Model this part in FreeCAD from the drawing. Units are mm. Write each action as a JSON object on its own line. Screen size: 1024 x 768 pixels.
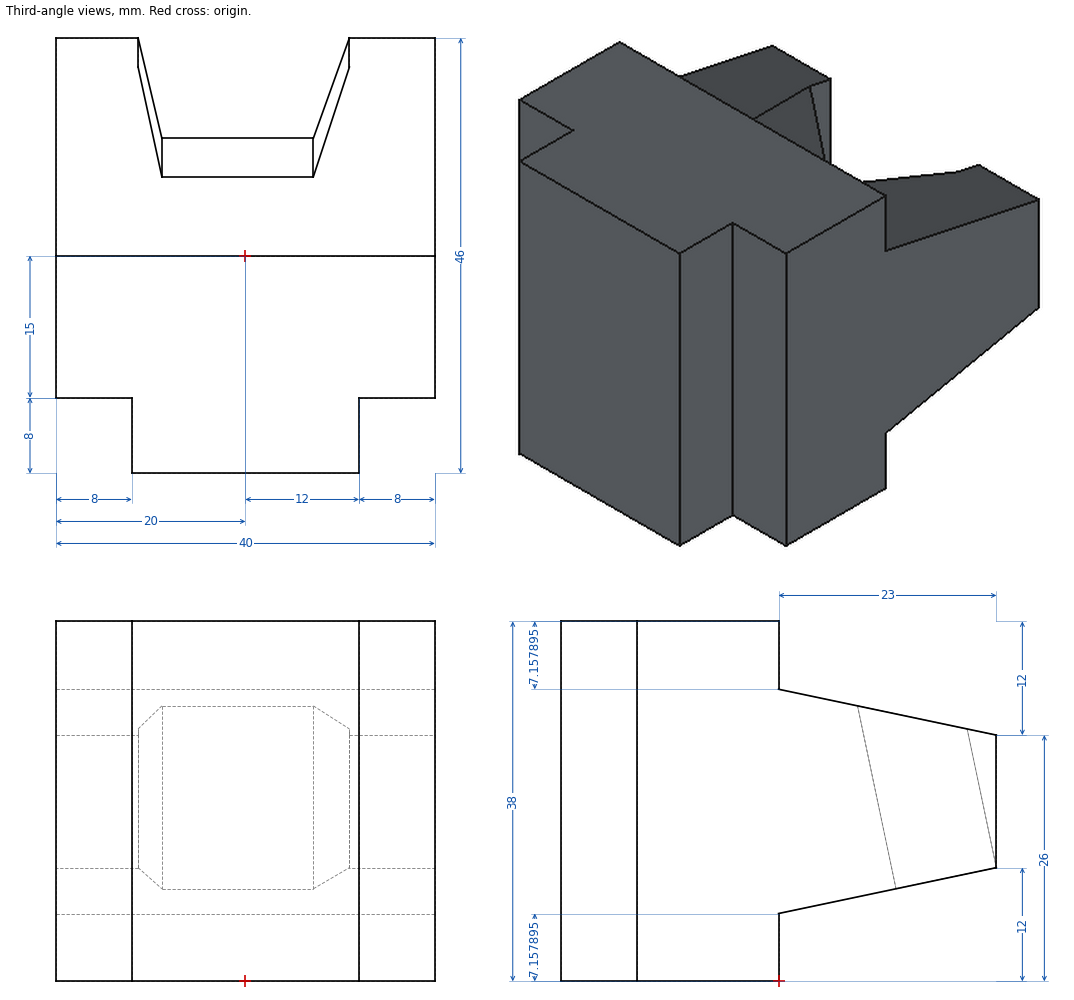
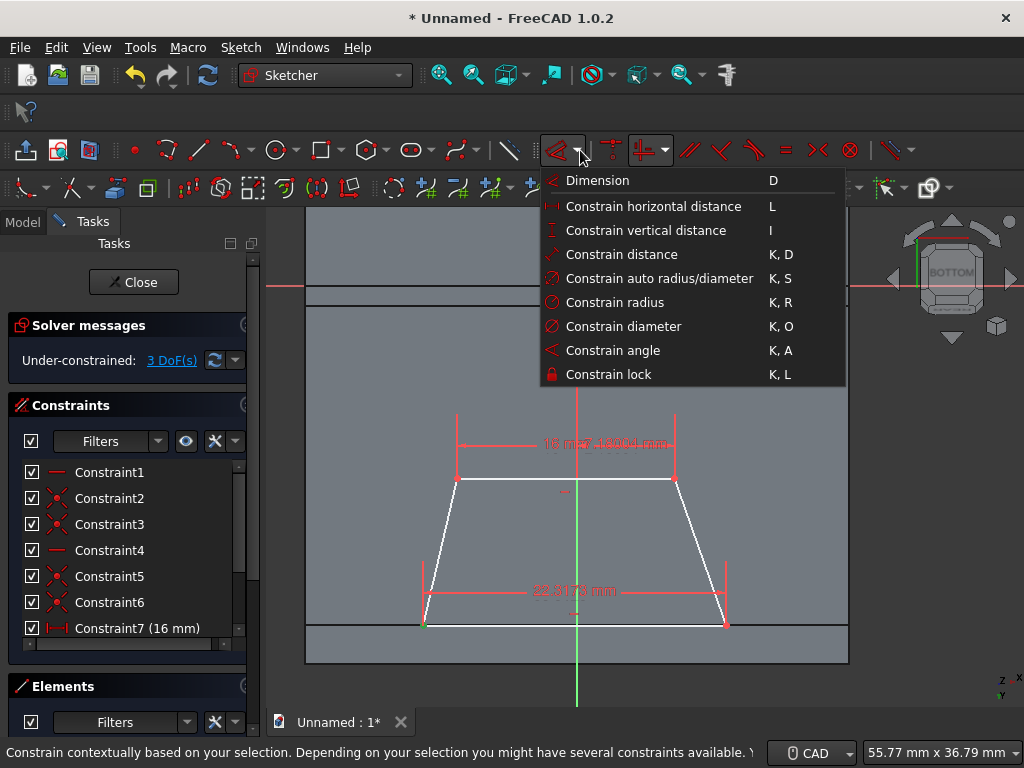
{"action": "left_click", "coordinate": [693, 206]}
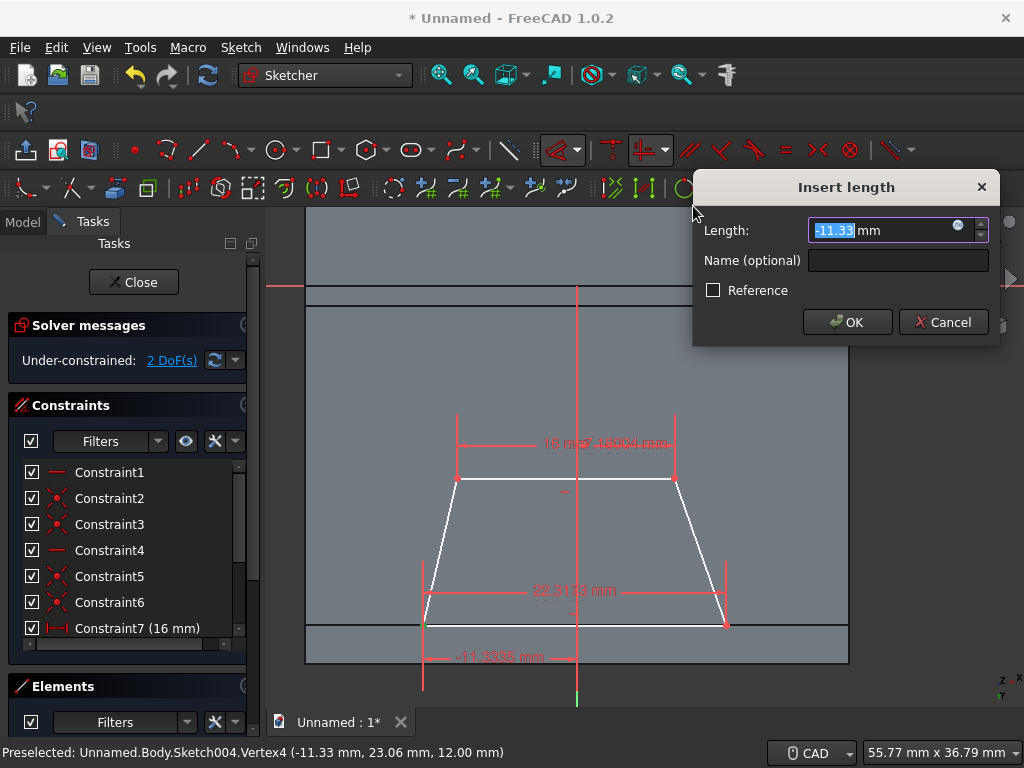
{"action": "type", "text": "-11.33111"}
{"action": "key", "text": "Return"}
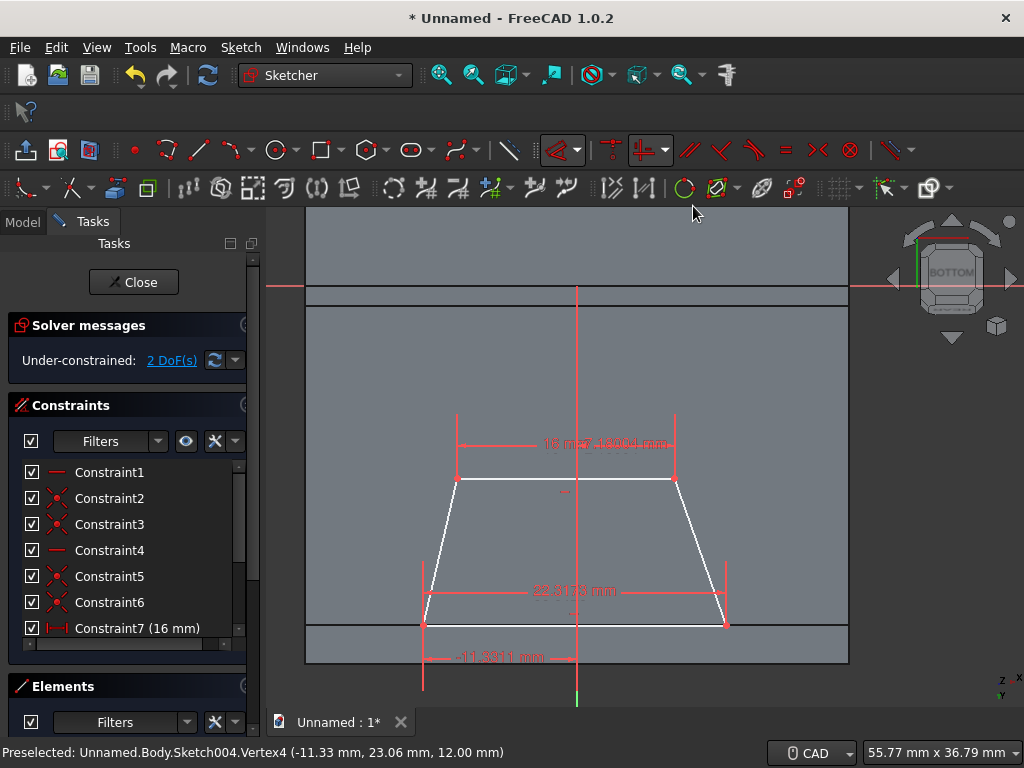
{"action": "left_click", "coordinate": [675, 479]}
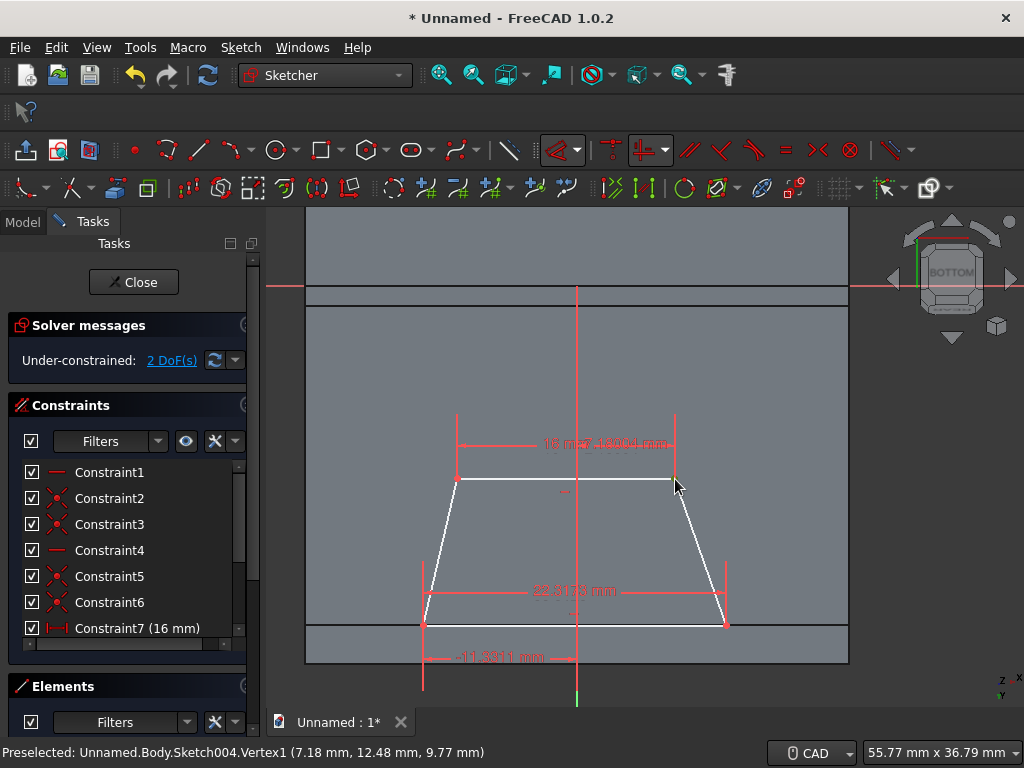
{"action": "key", "text": "i"}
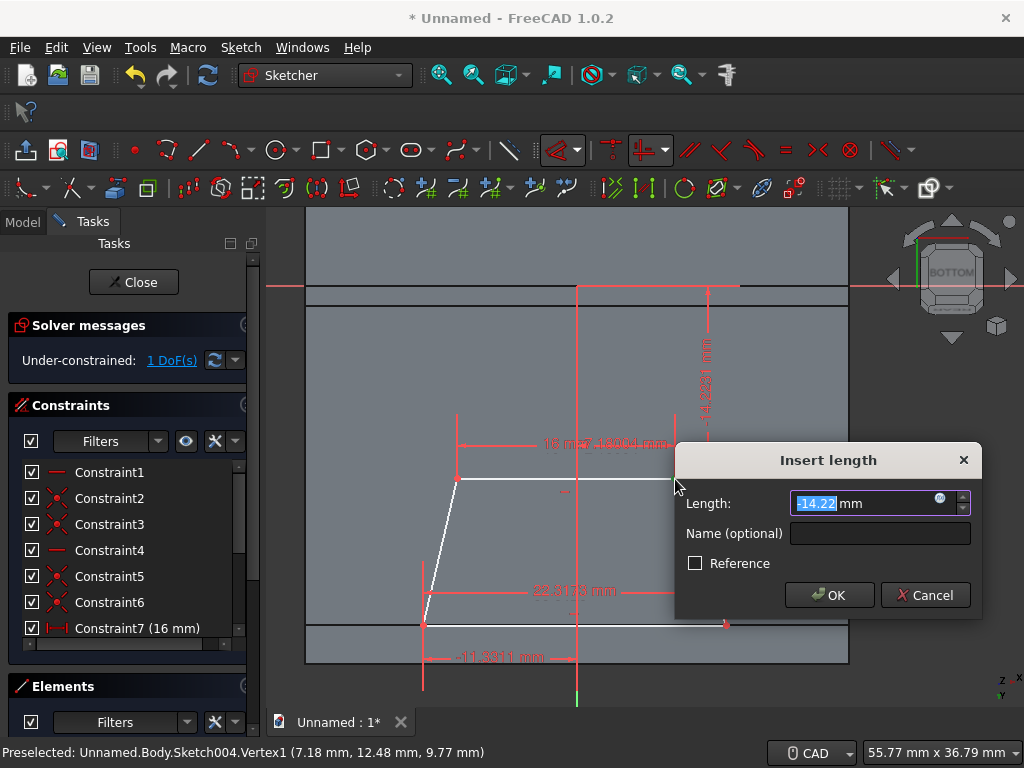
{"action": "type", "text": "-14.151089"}
{"action": "key", "text": "Return"}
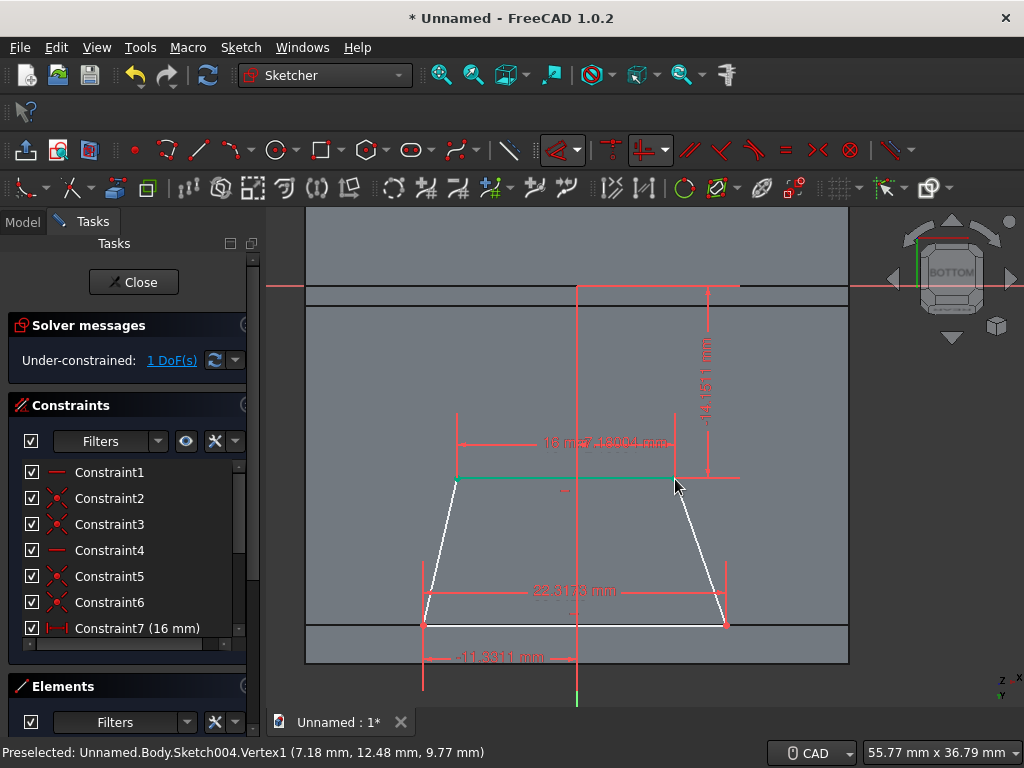
{"action": "left_click", "coordinate": [423, 626]}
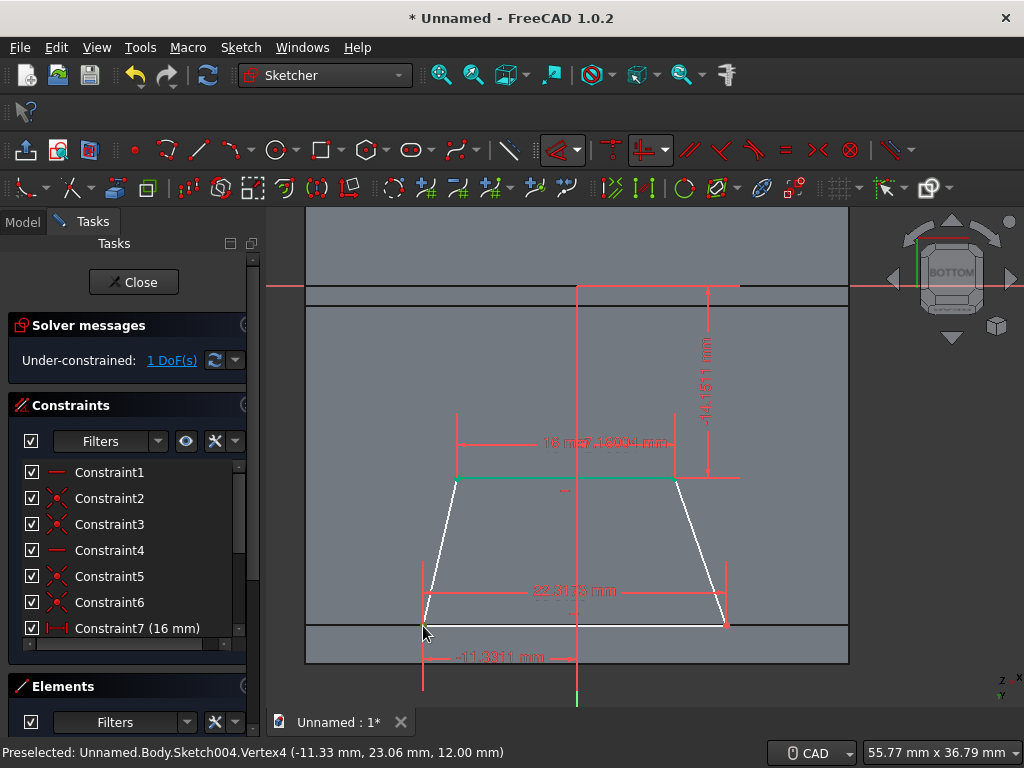
{"action": "left_click", "coordinate": [580, 150]}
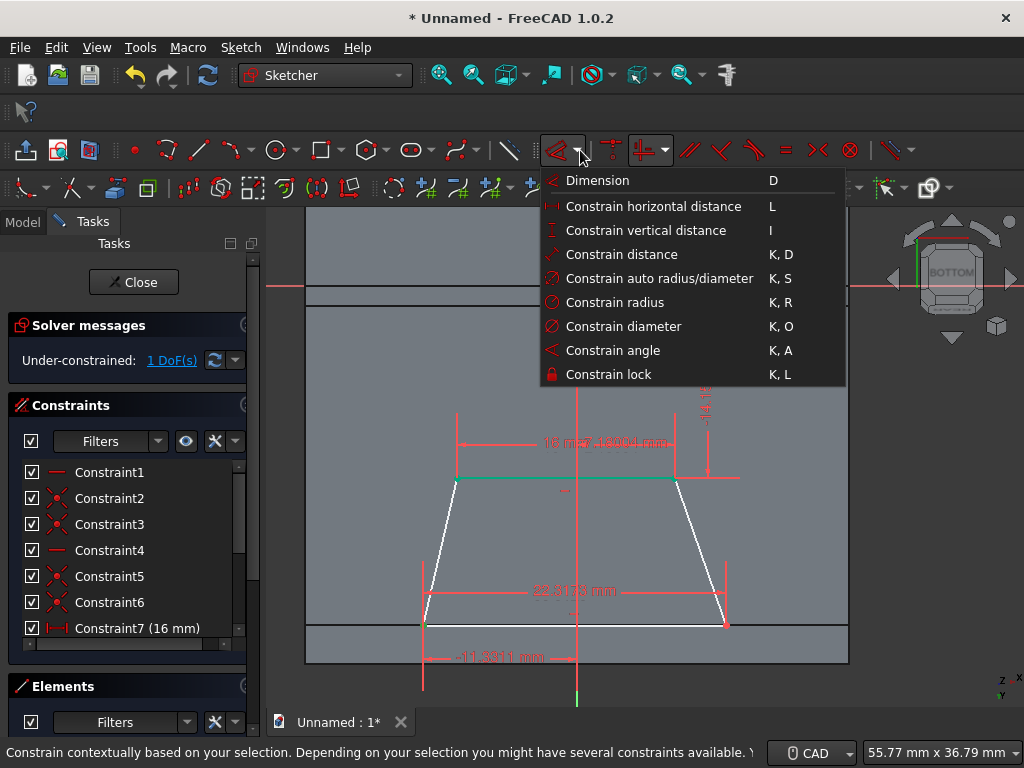
{"action": "left_click", "coordinate": [693, 230]}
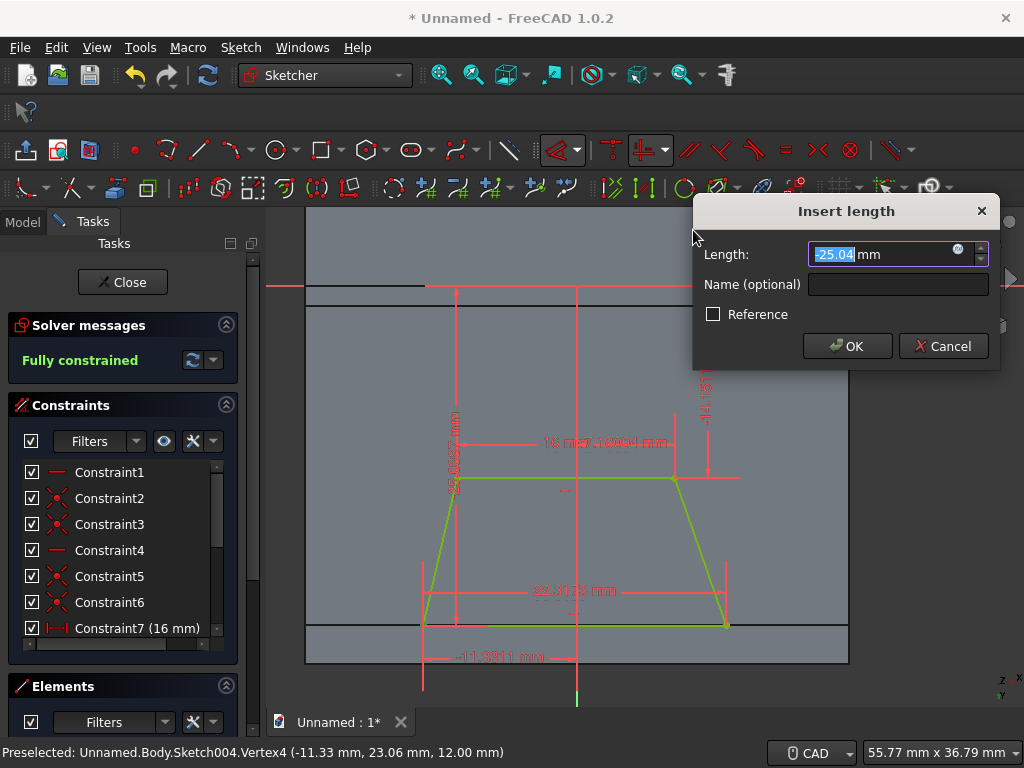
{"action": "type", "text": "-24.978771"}
{"action": "key", "text": "Return"}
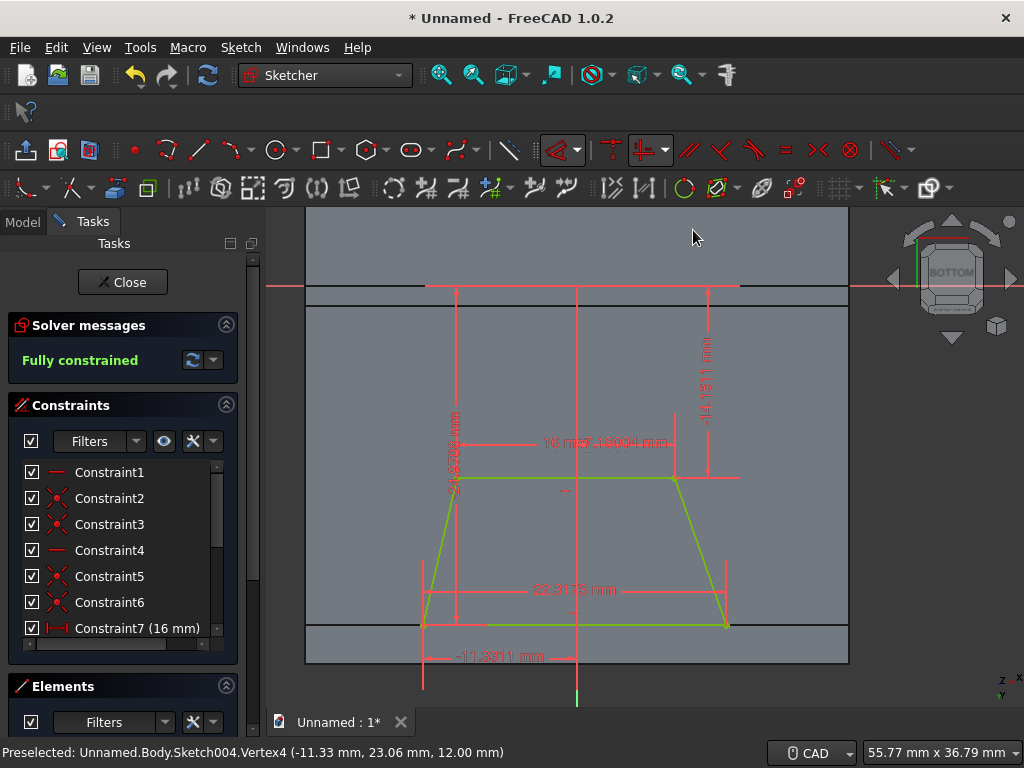
{"action": "left_click", "coordinate": [123, 282]}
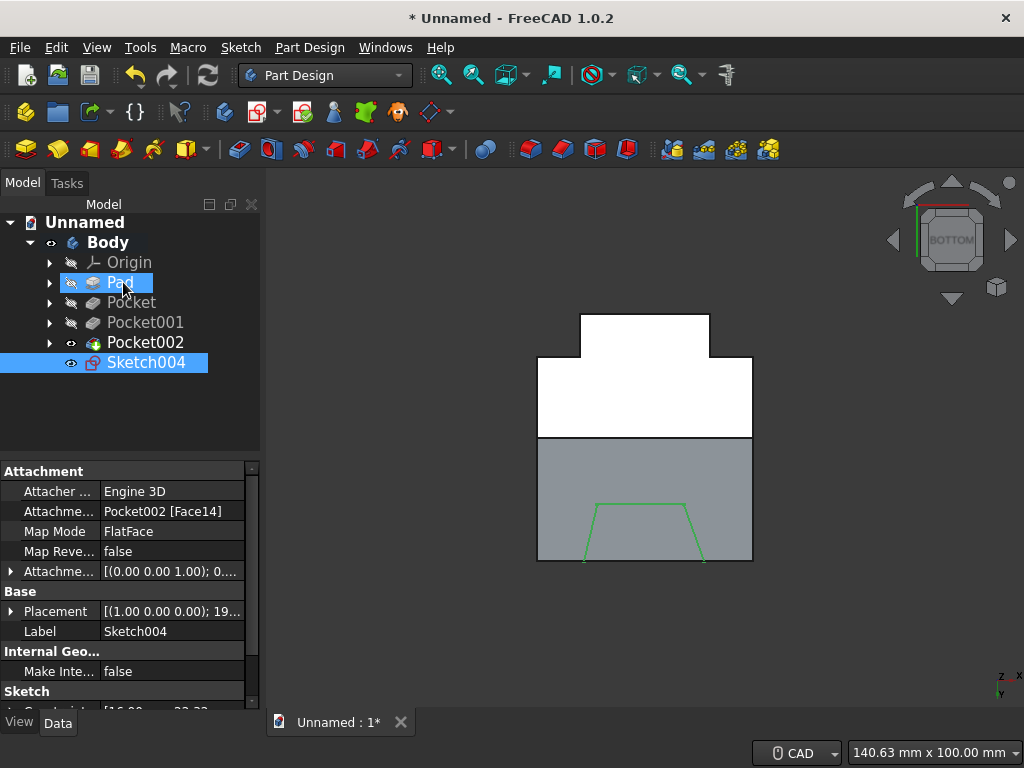
{"action": "left_click", "coordinate": [240, 150]}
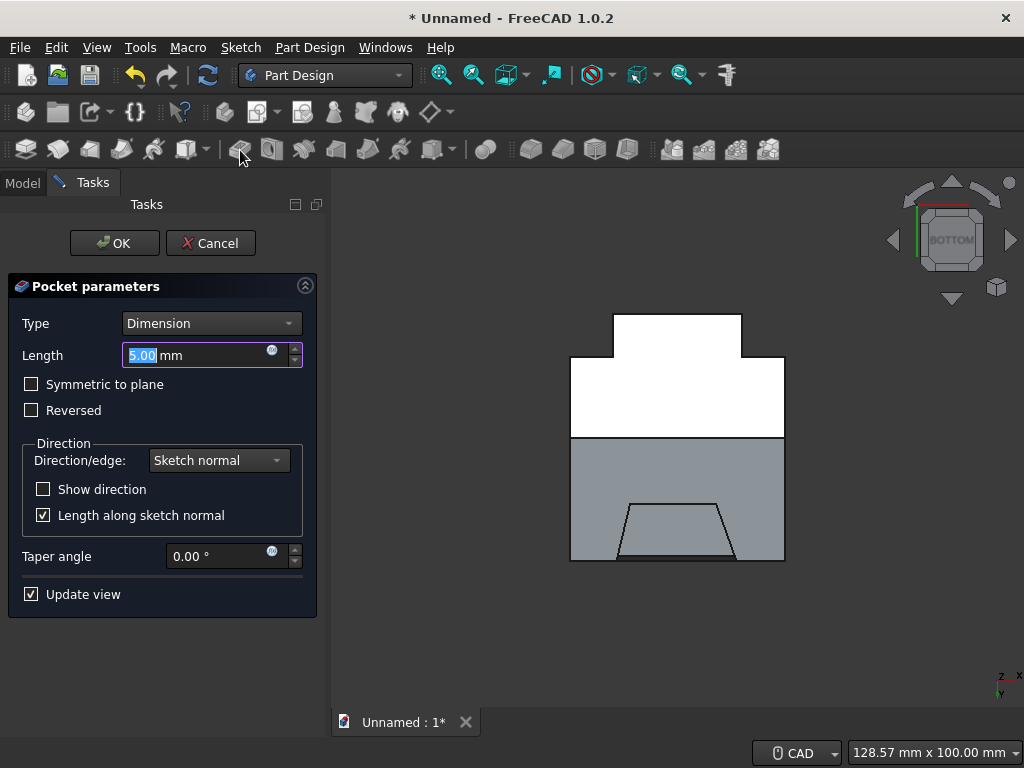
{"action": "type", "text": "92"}
{"action": "key", "text": "Tab"}